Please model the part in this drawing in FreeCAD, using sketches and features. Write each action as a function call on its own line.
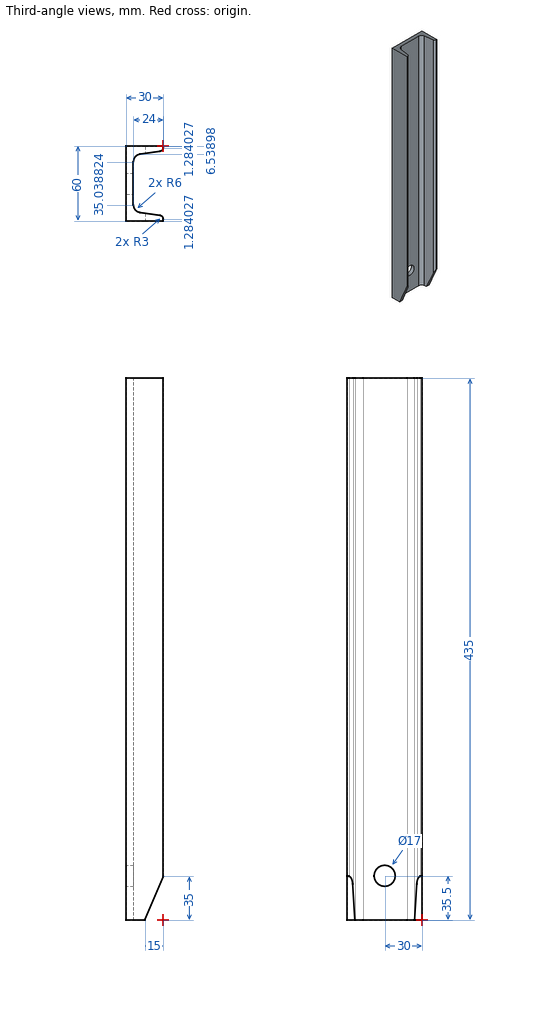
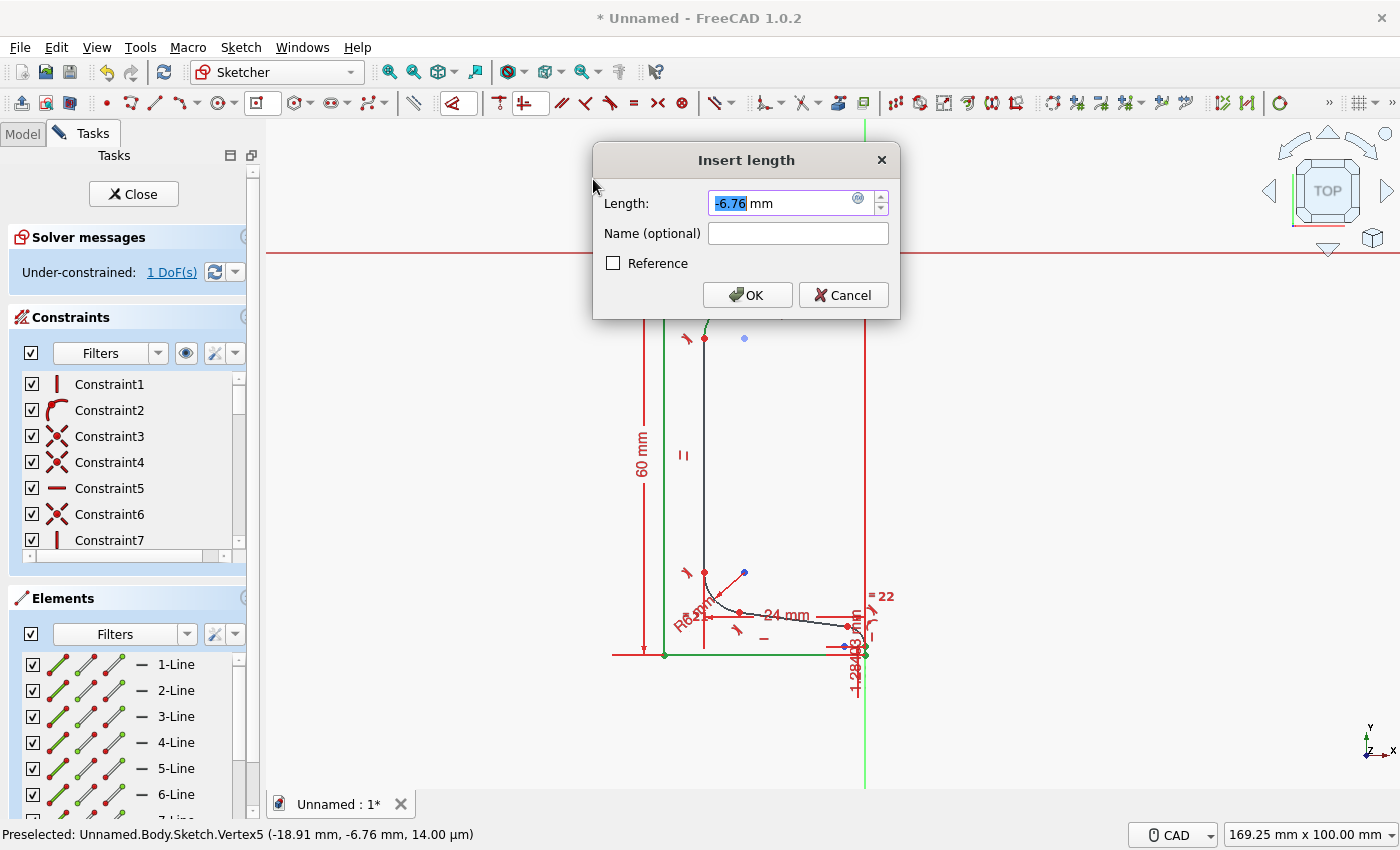
text(-6.53898)
key(Return)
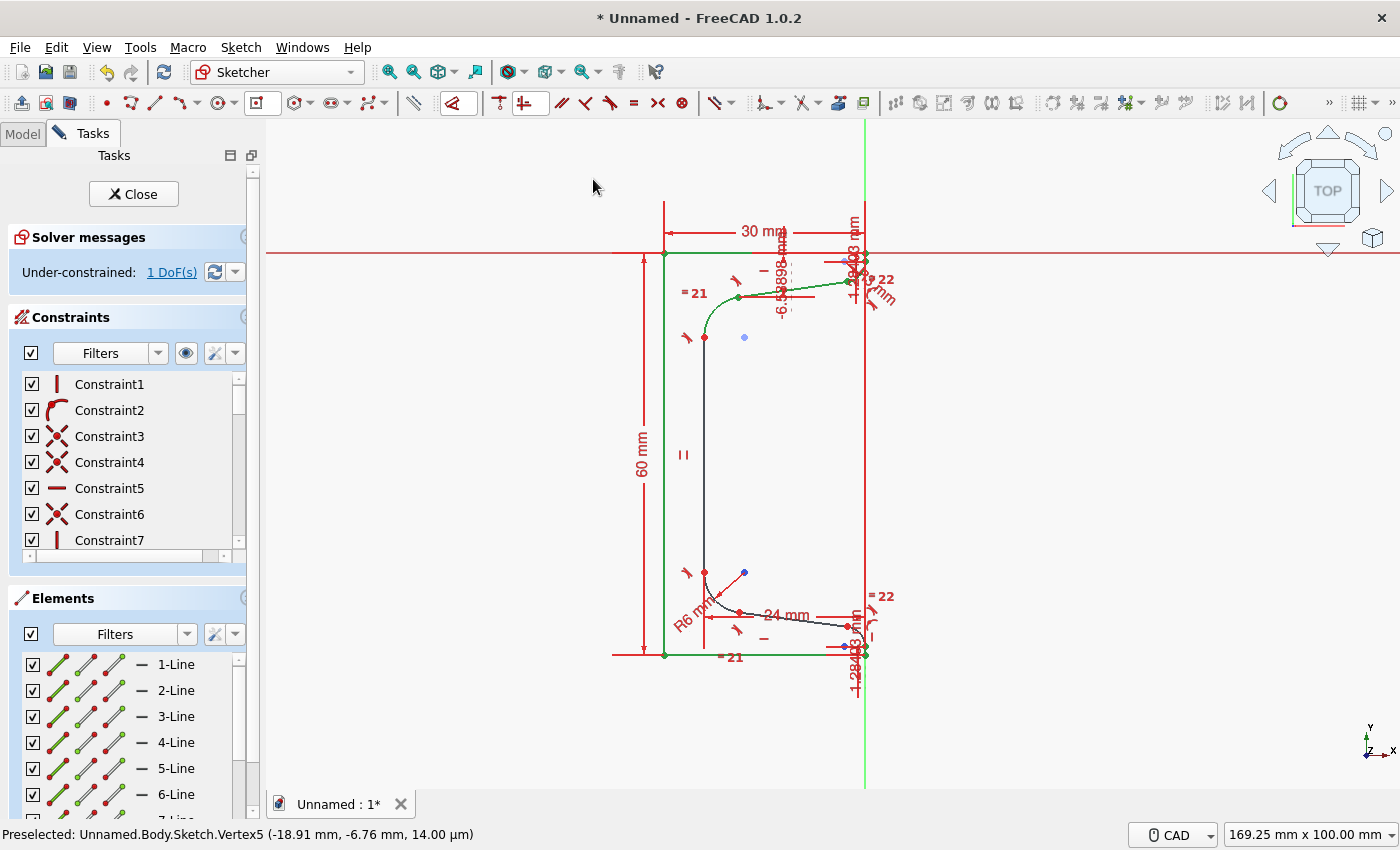
click(704, 502)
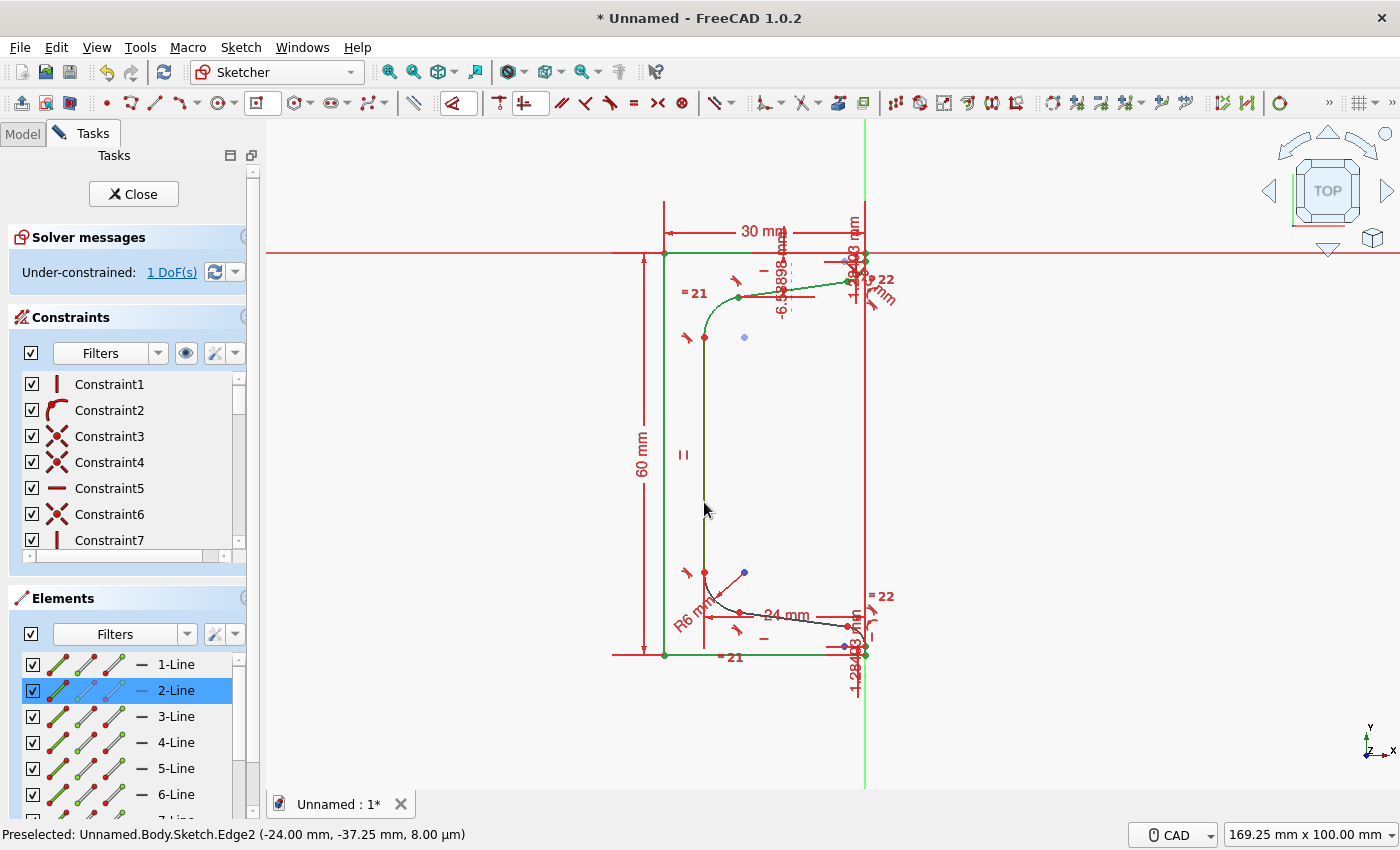
key(i)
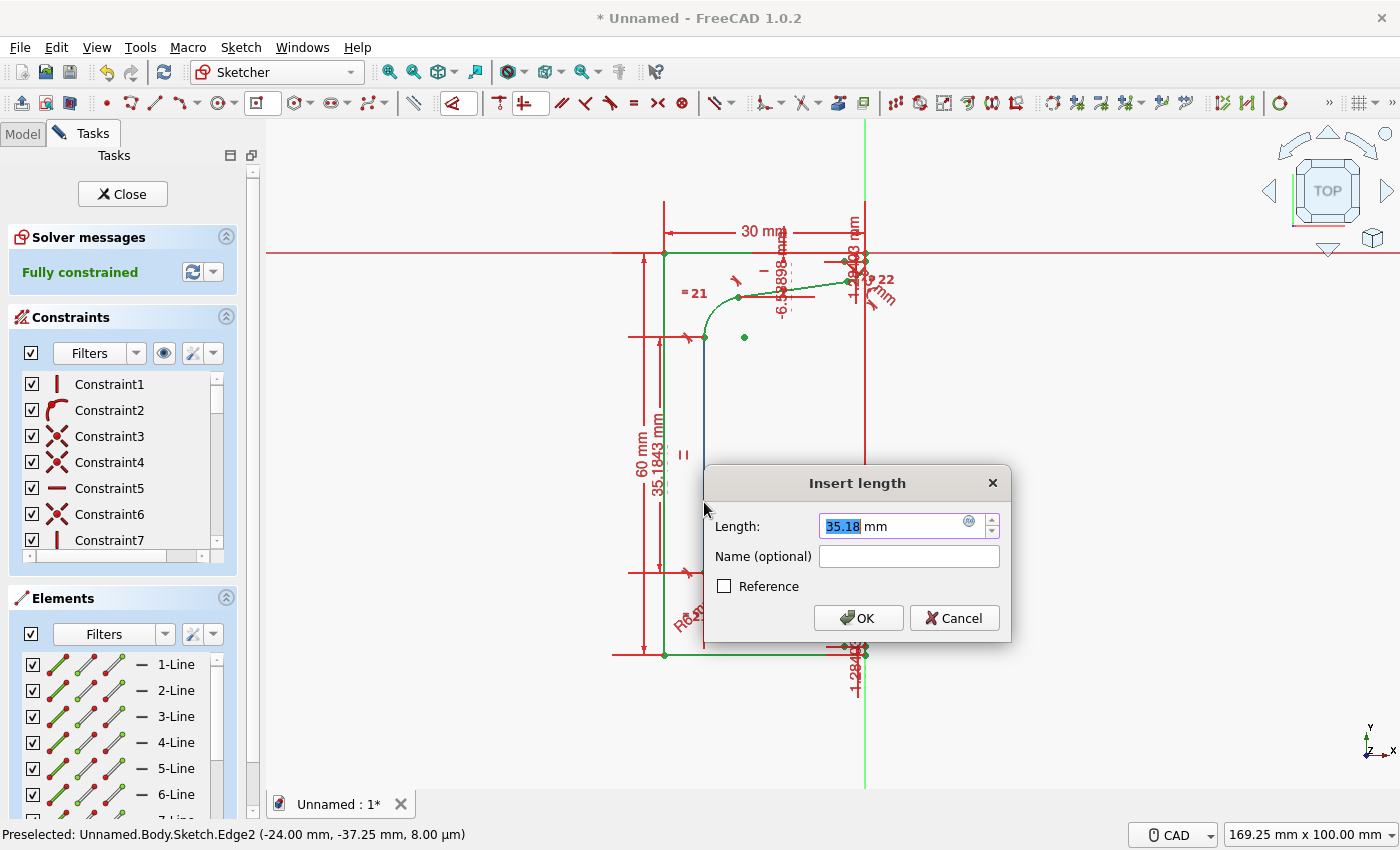
text(35.038824)
key(Return)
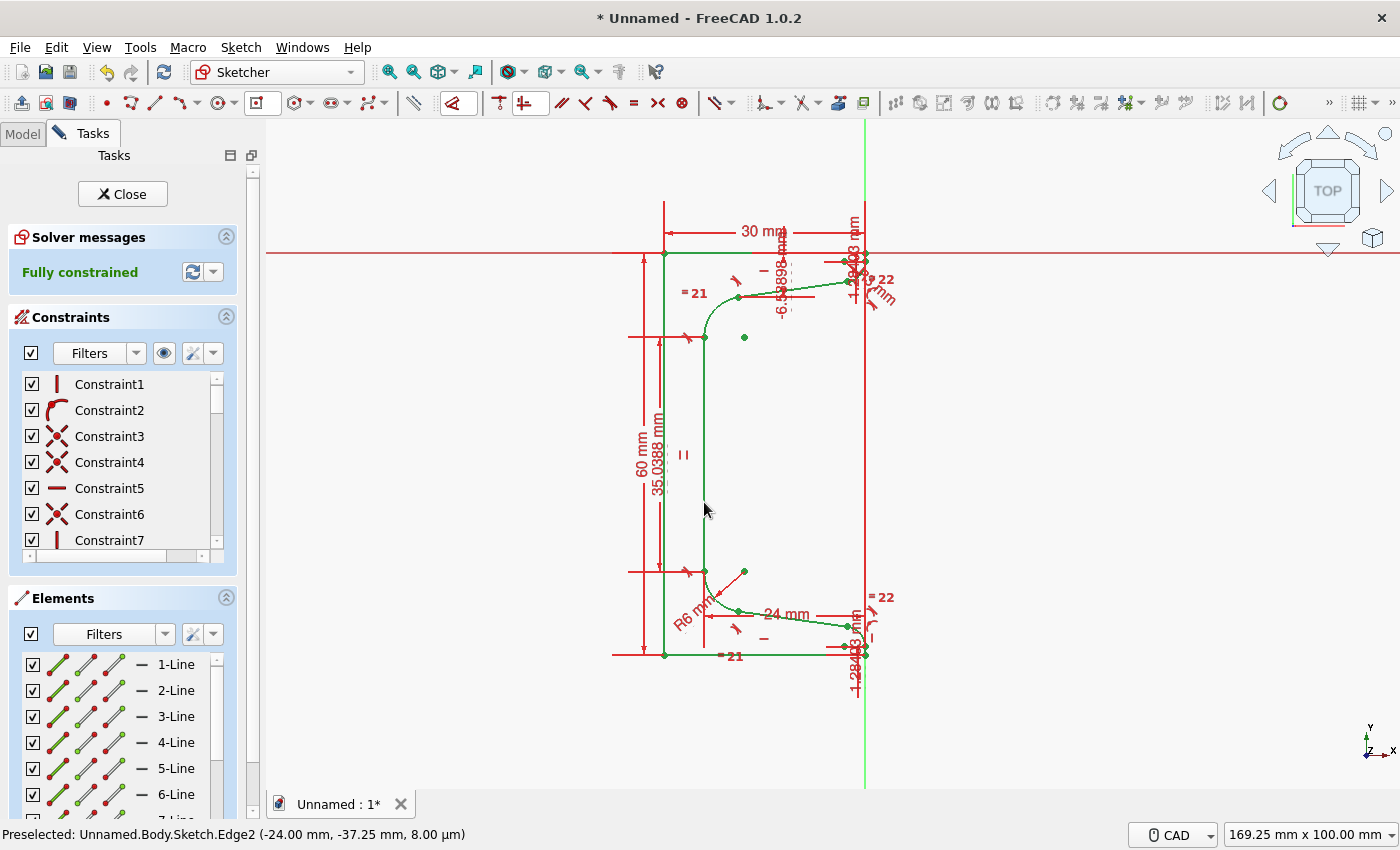
click(123, 194)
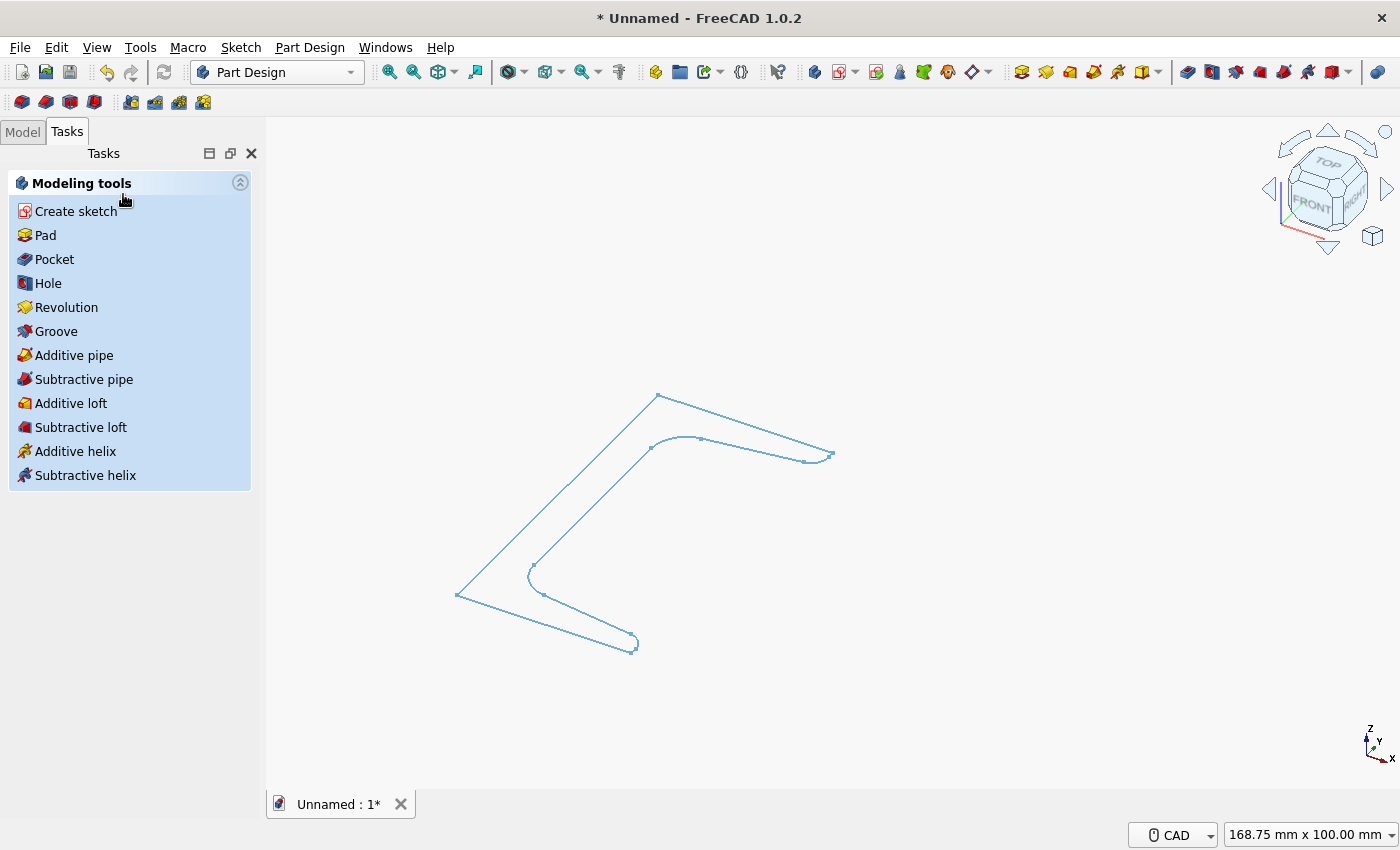
click(1022, 72)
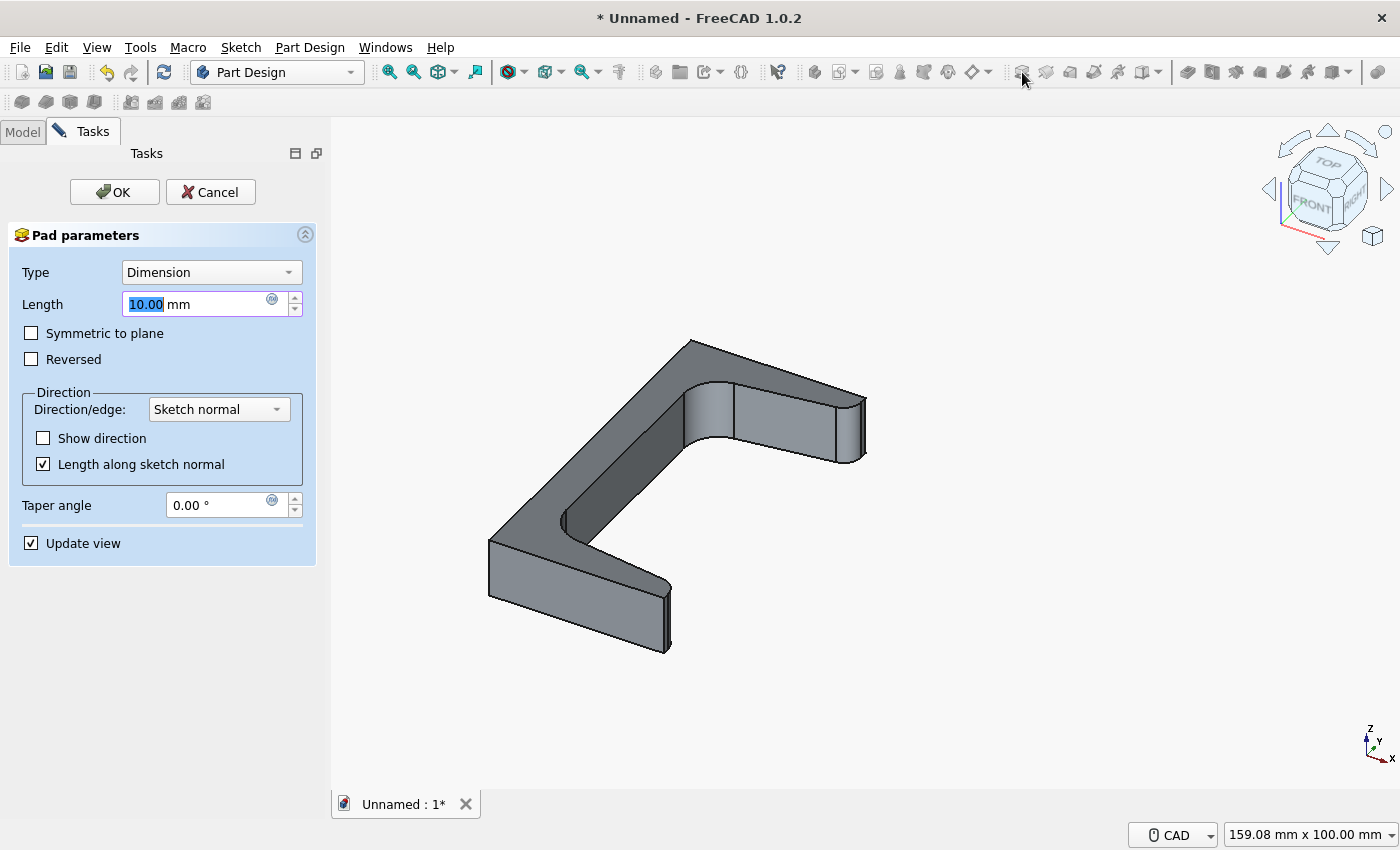
text(435)
key(Tab)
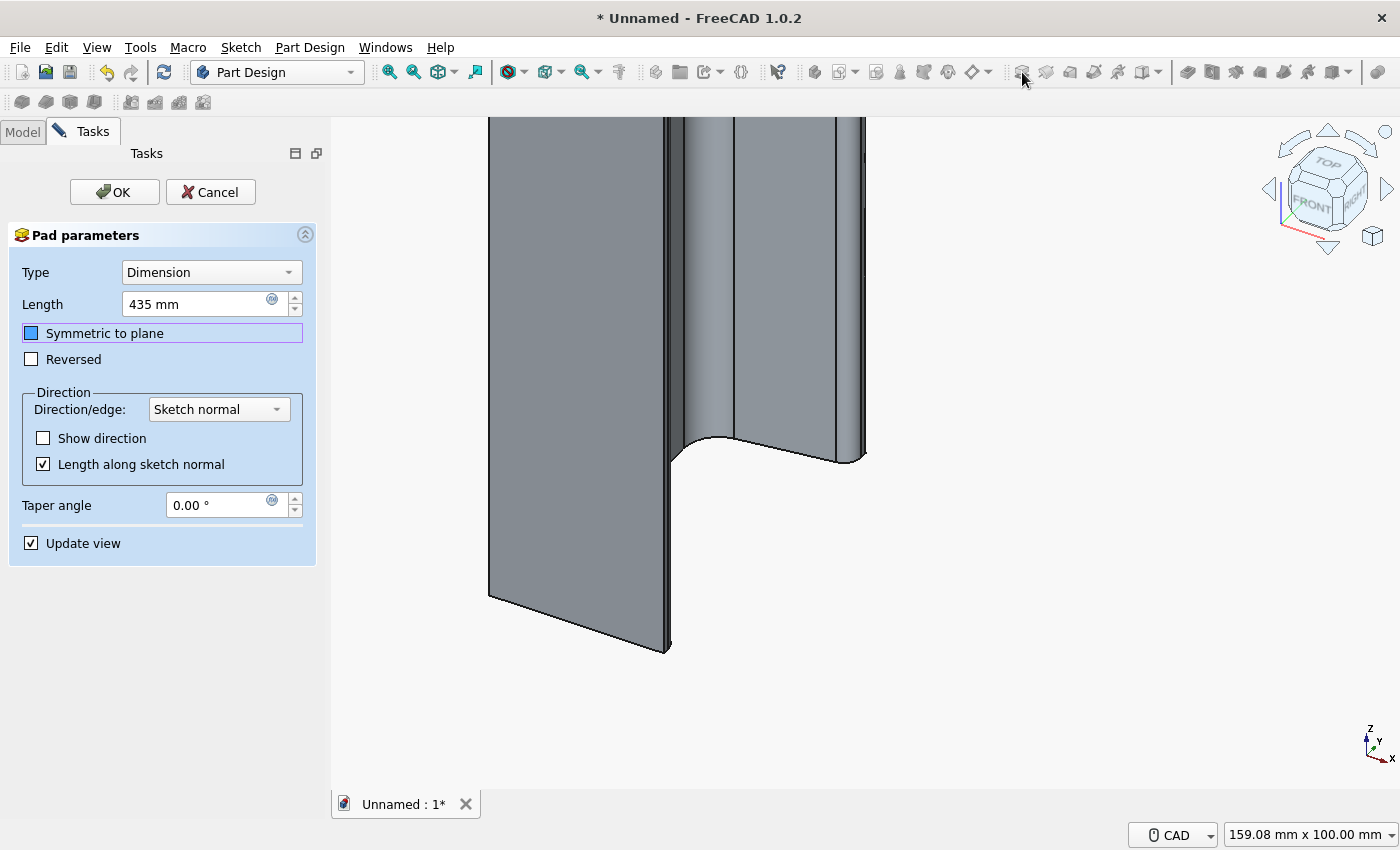
click(115, 192)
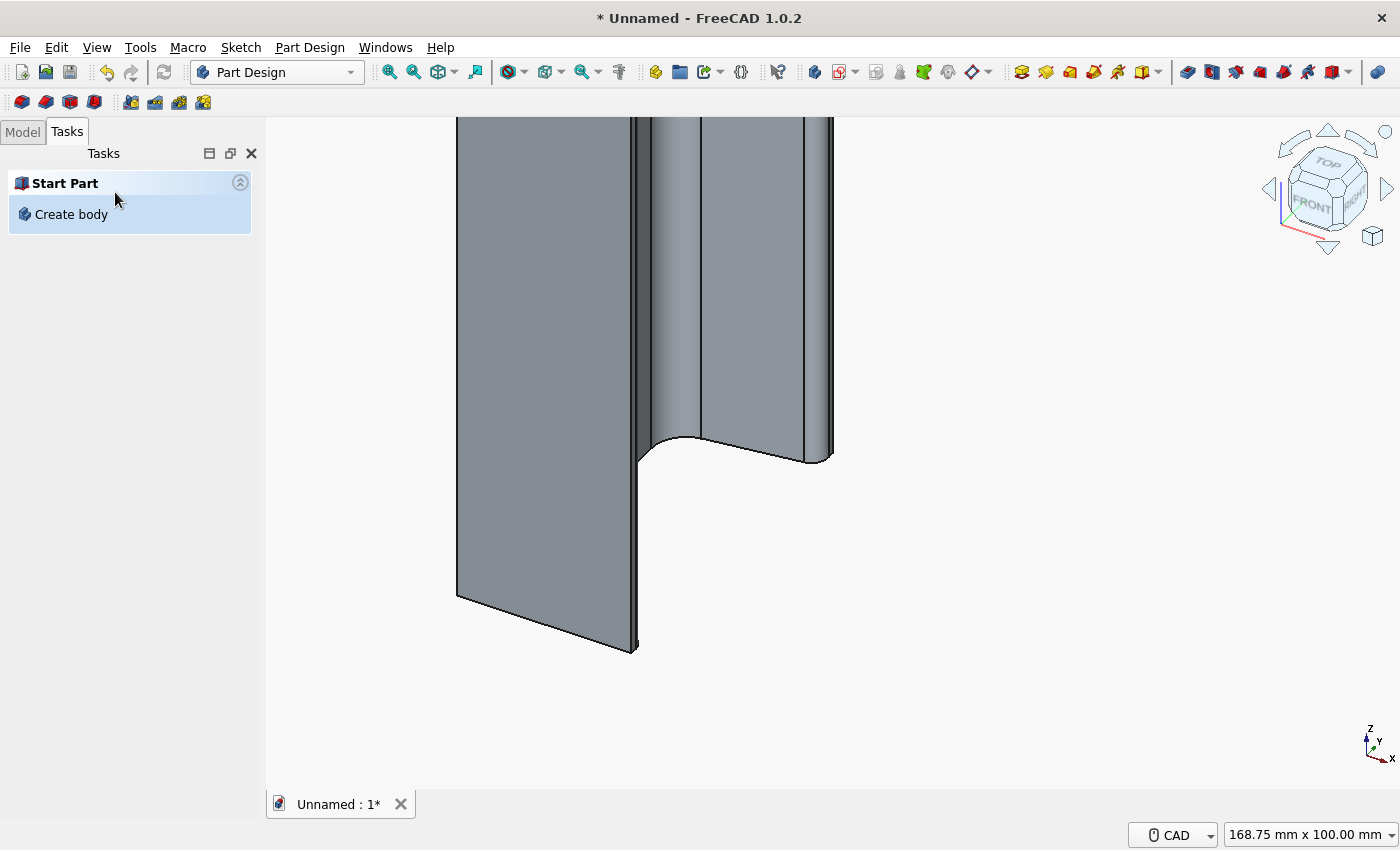
click(390, 72)